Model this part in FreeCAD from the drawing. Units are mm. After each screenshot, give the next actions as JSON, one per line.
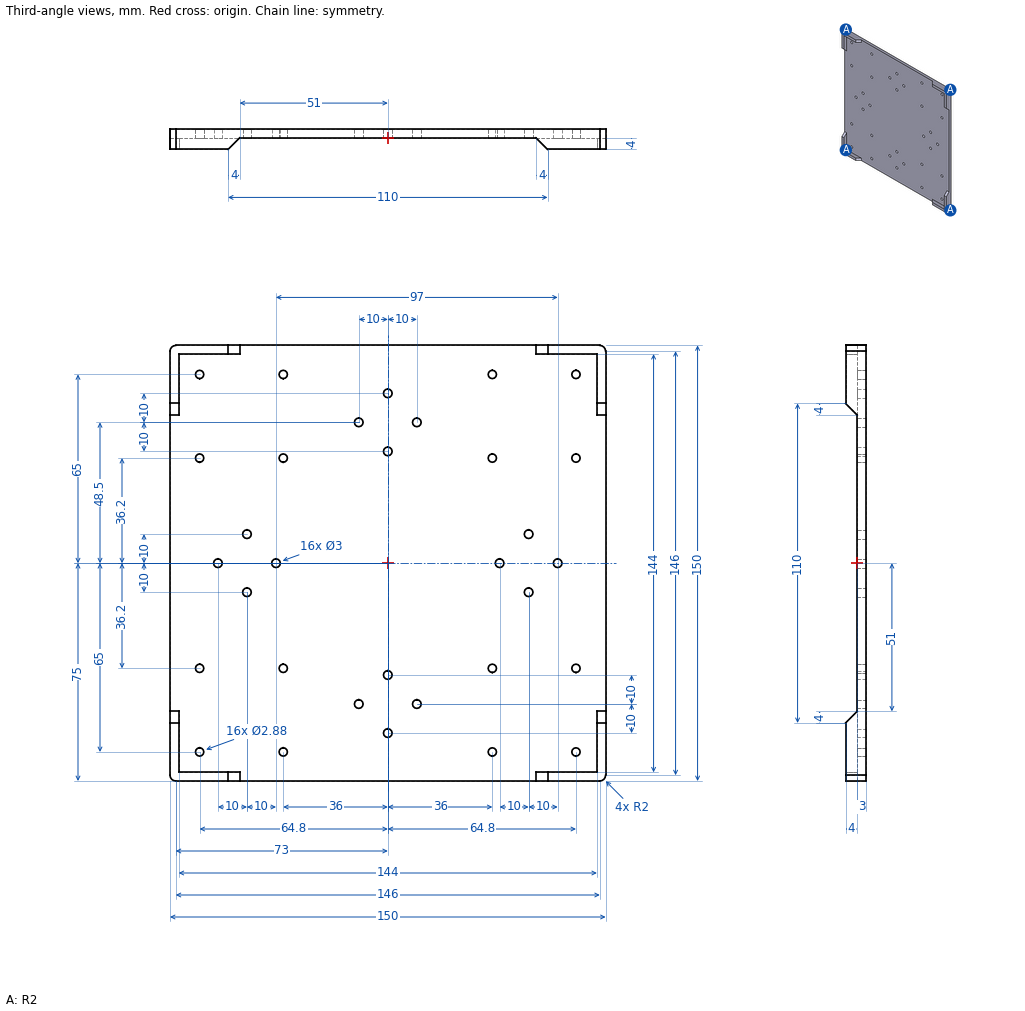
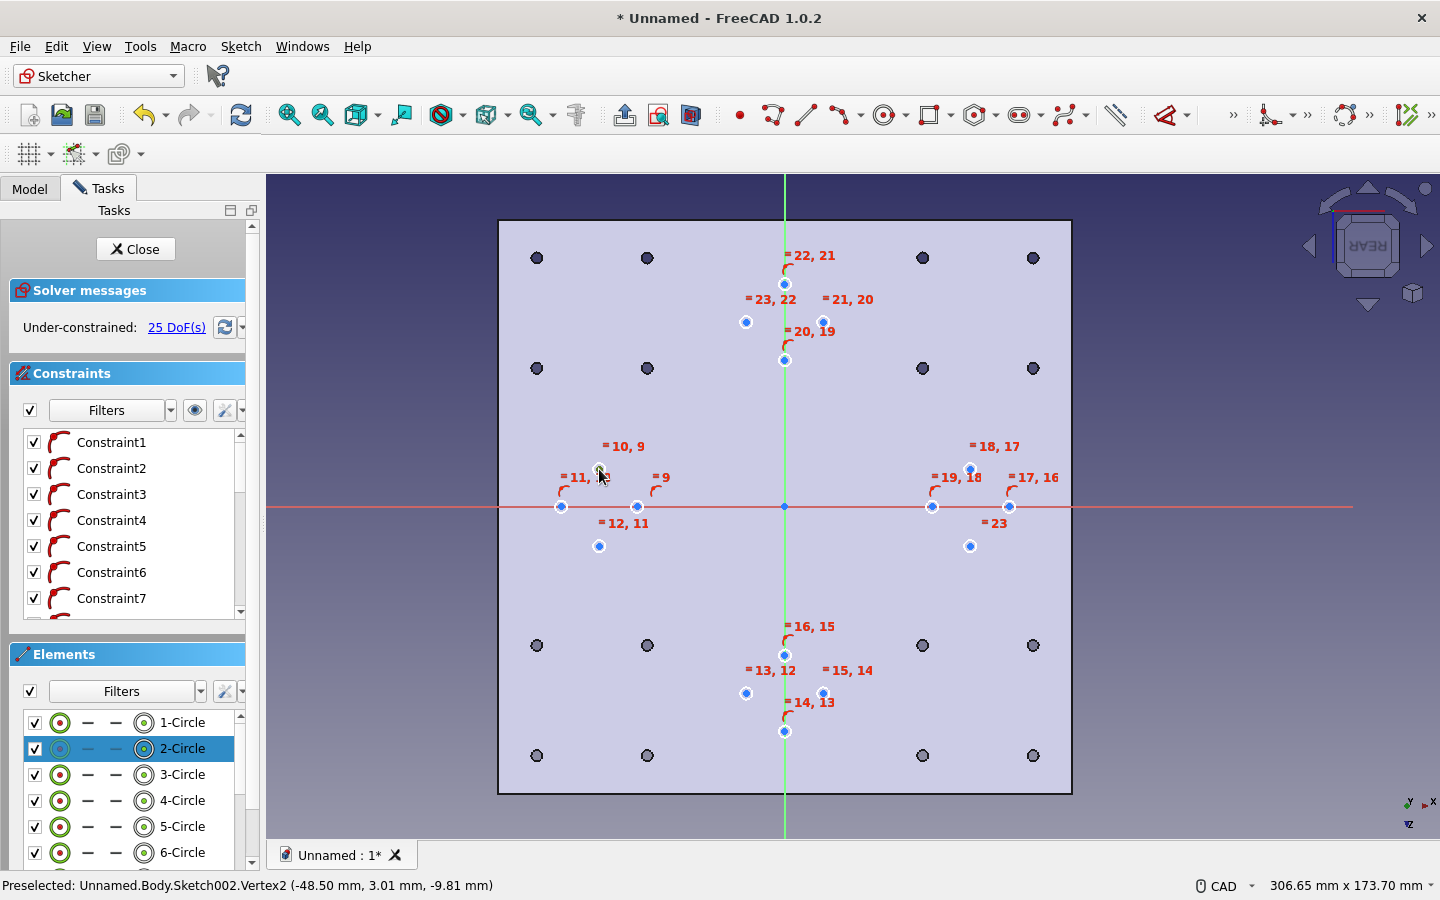
{"action": "left_click", "coordinate": [599, 546]}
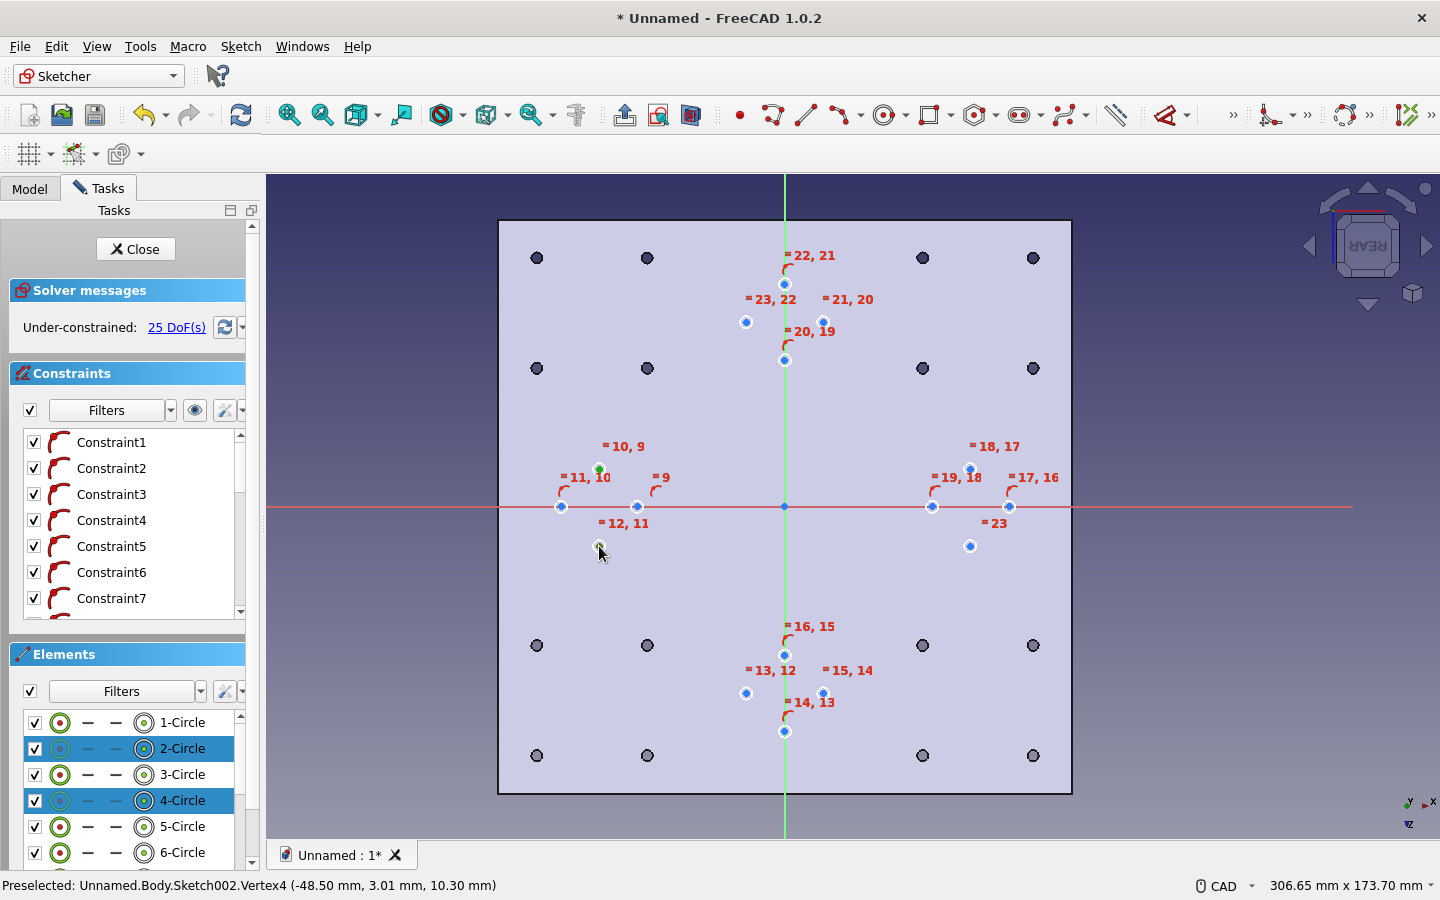
{"action": "key", "text": "v"}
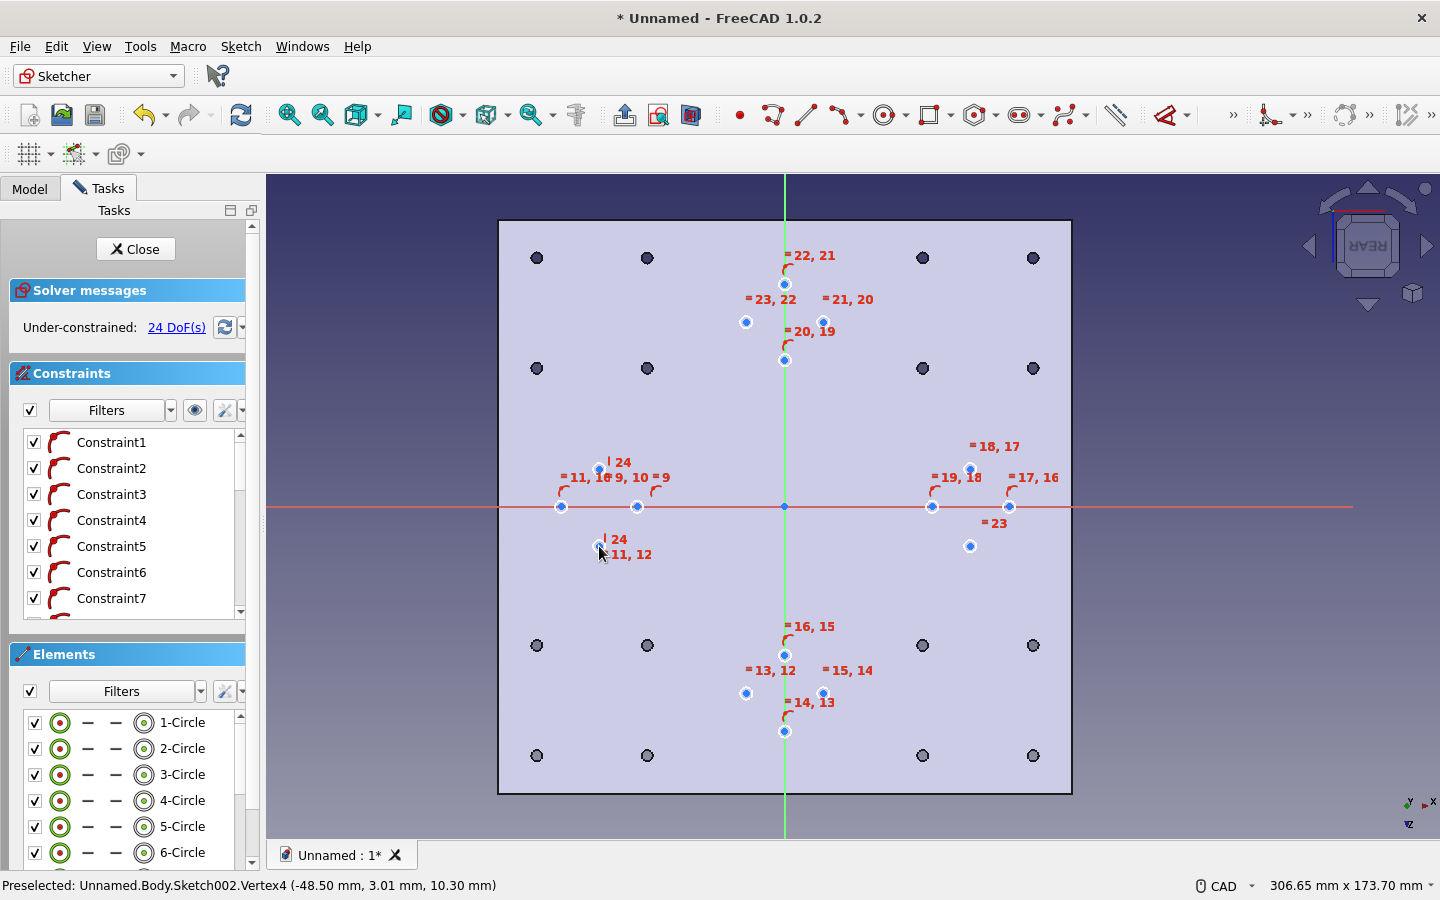
{"action": "left_click", "coordinate": [746, 694]}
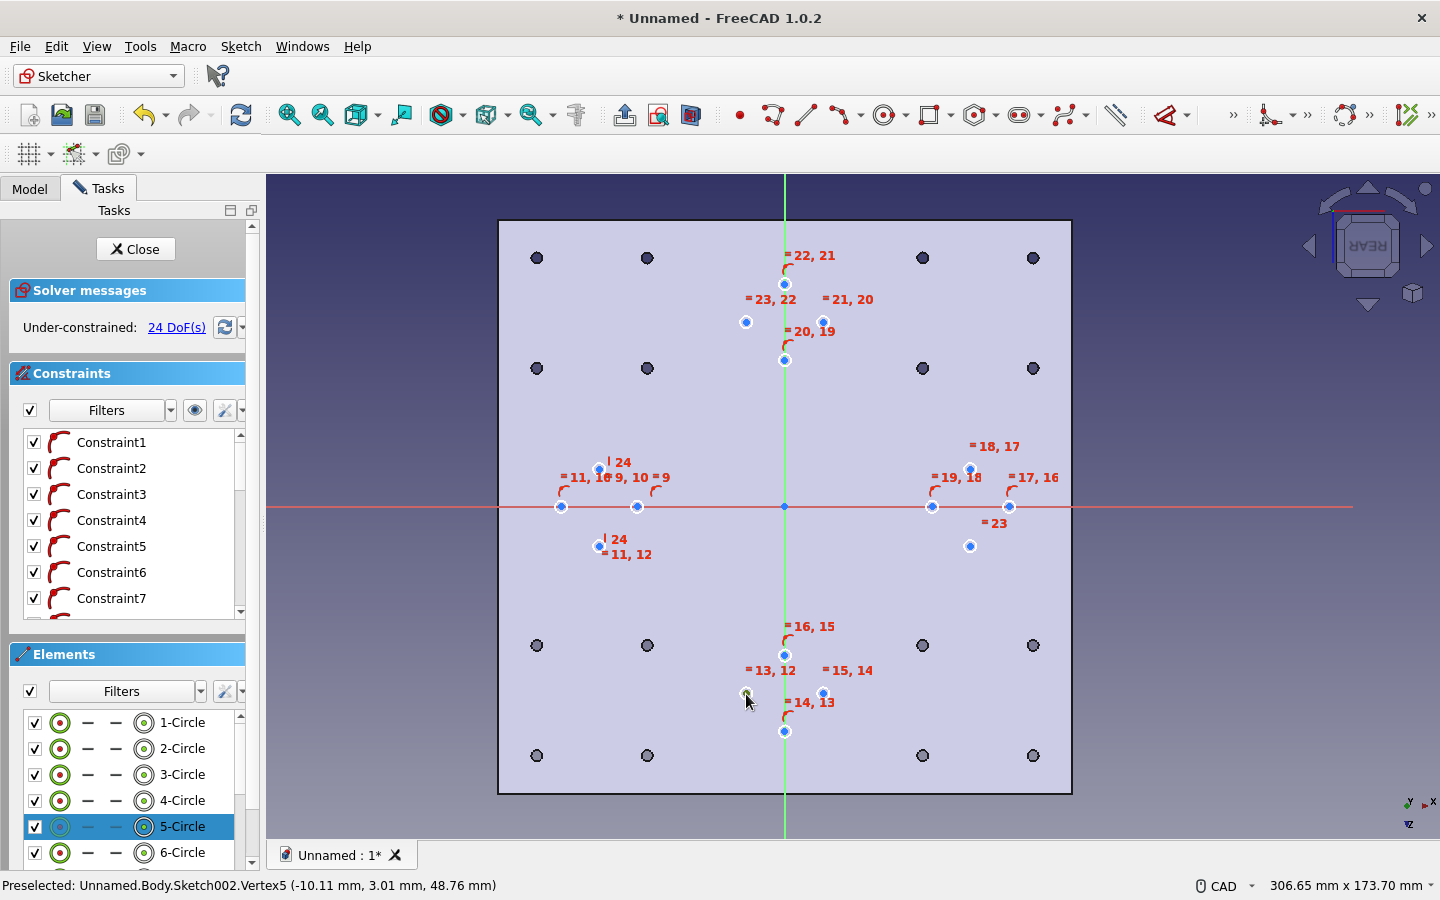
{"action": "left_click", "coordinate": [823, 694]}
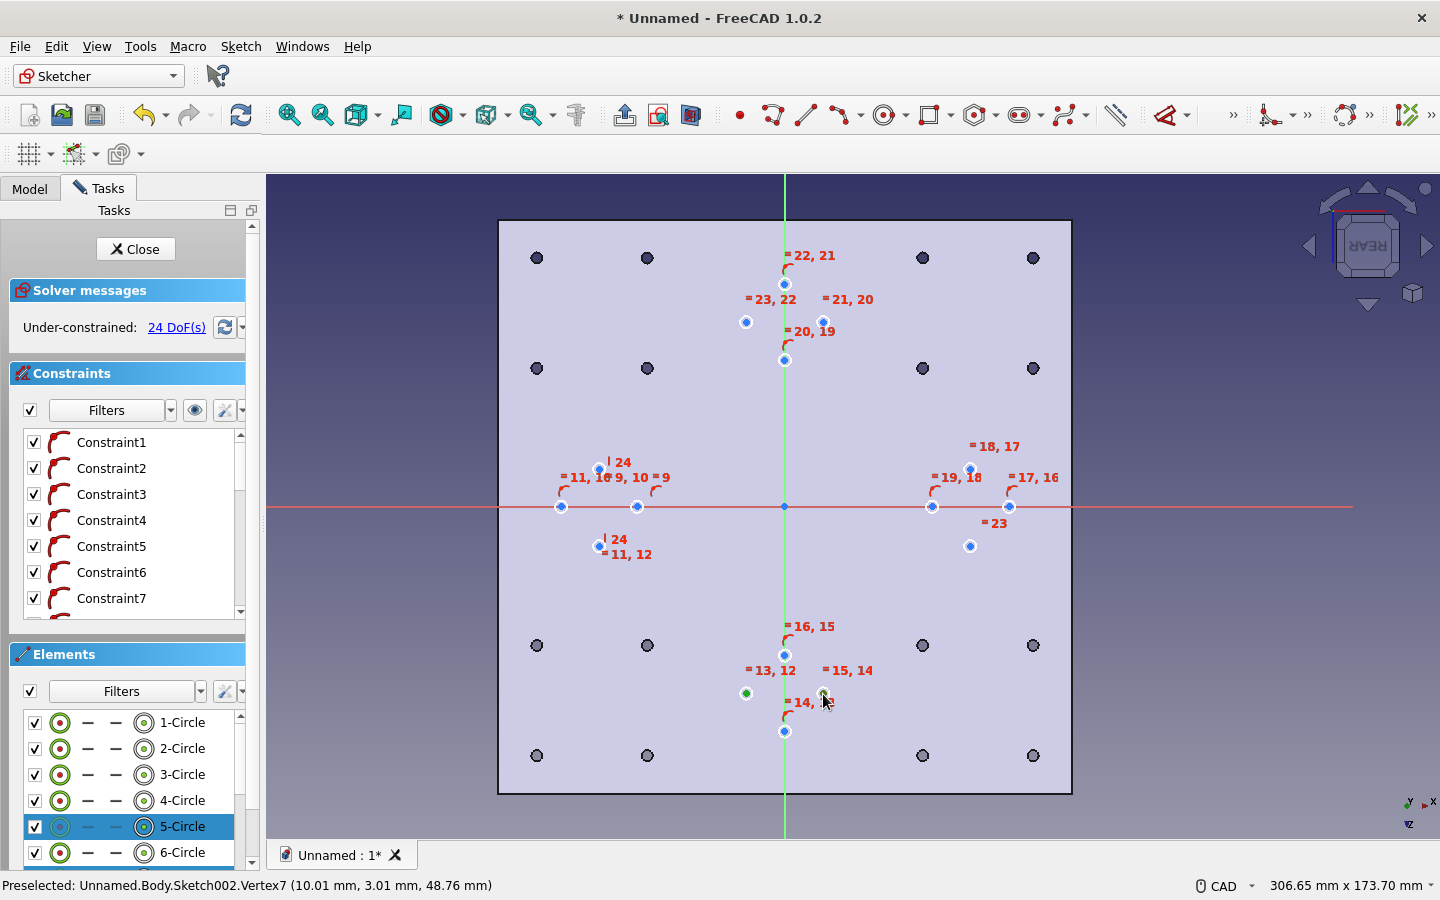
{"action": "key", "text": "h"}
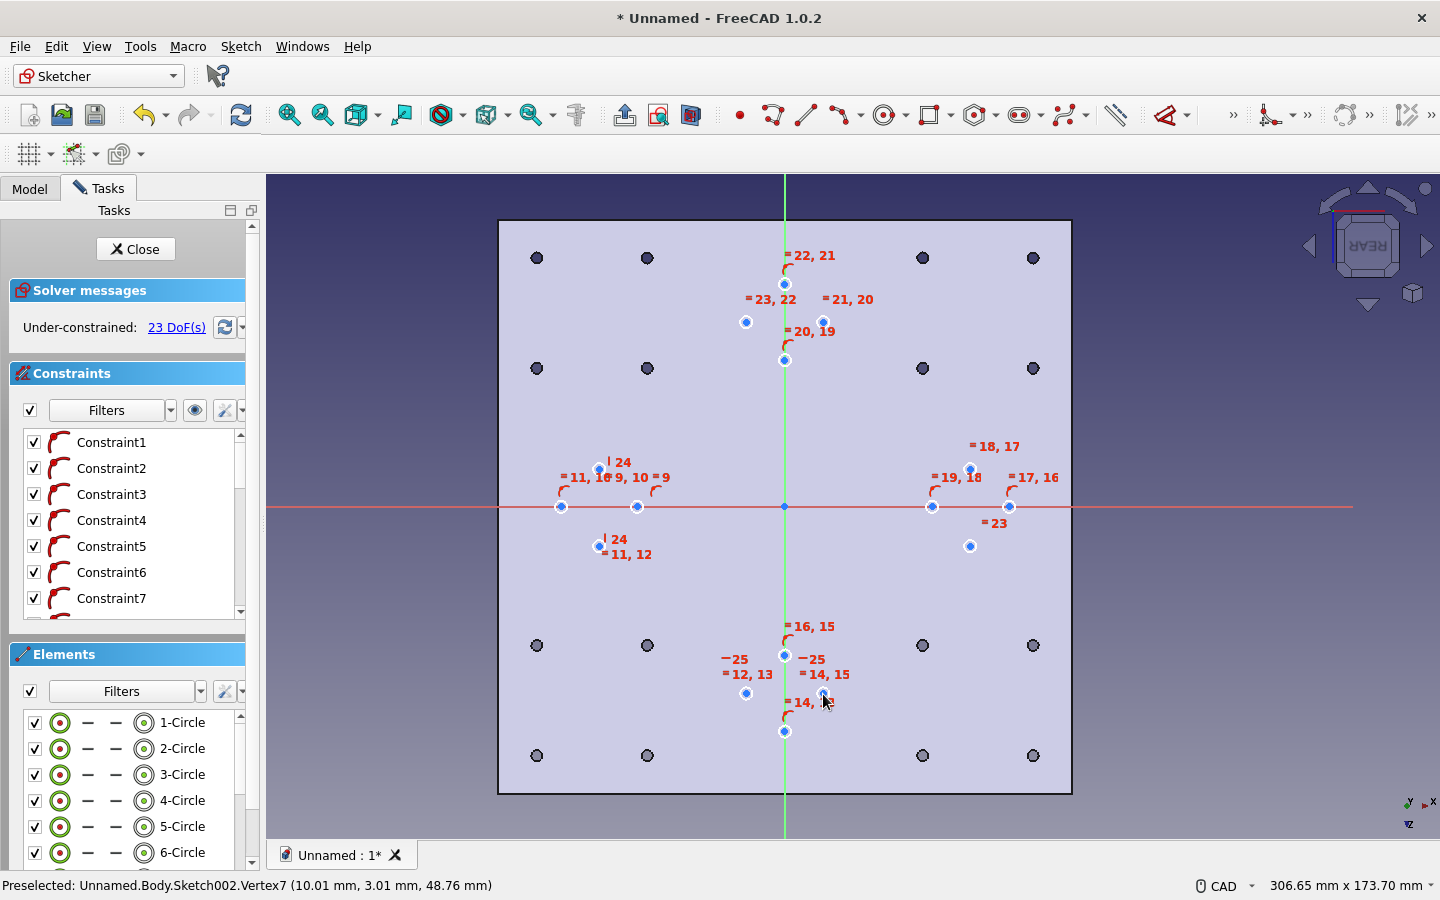
{"action": "left_click", "coordinate": [823, 322]}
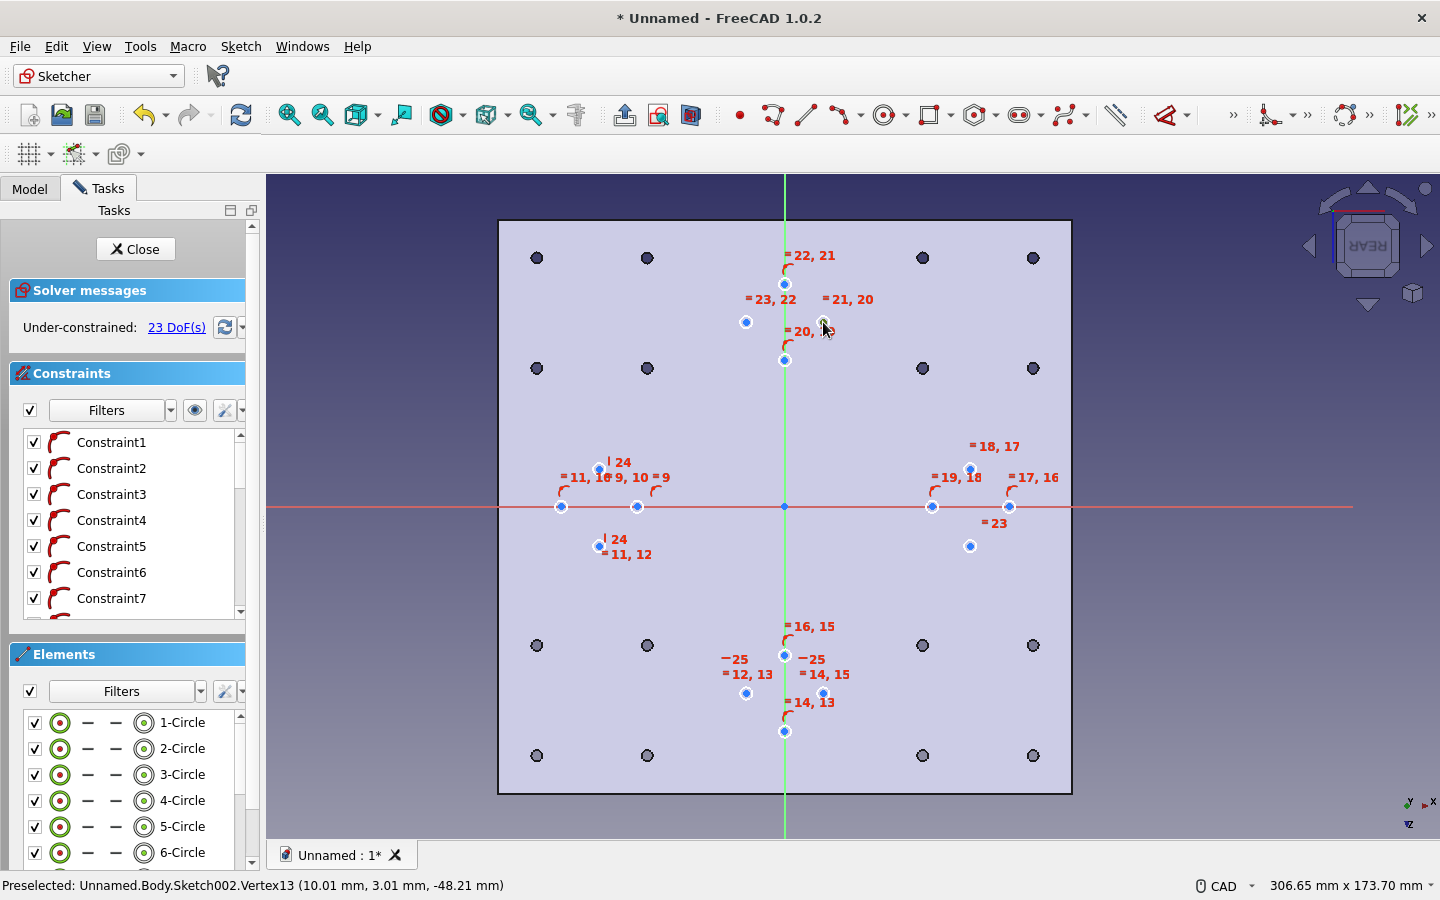
{"action": "left_click", "coordinate": [746, 322]}